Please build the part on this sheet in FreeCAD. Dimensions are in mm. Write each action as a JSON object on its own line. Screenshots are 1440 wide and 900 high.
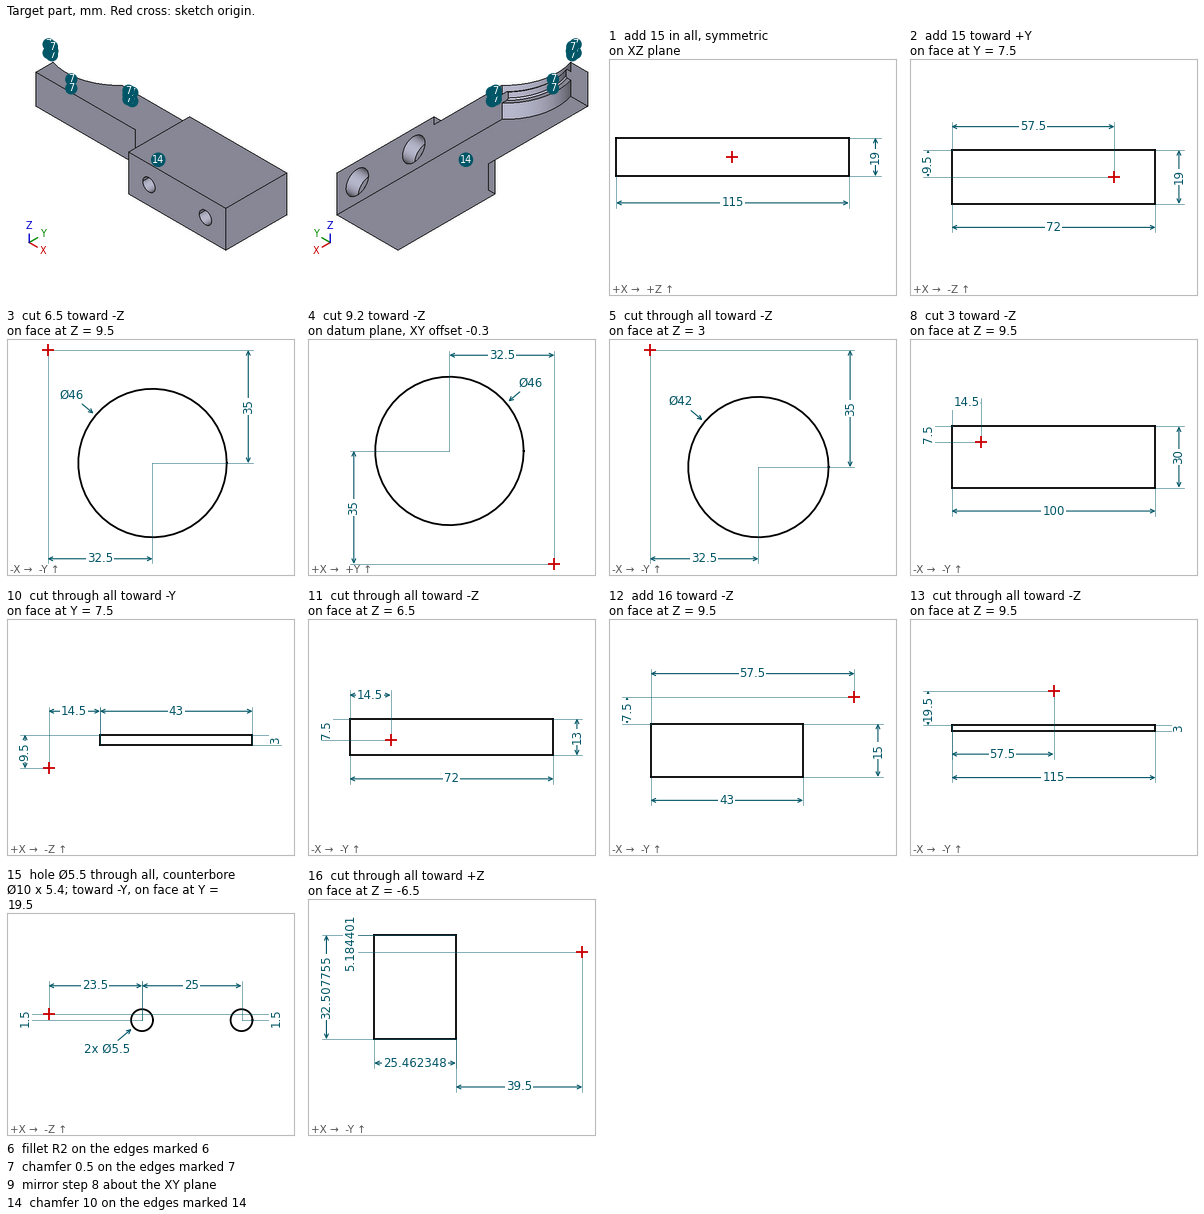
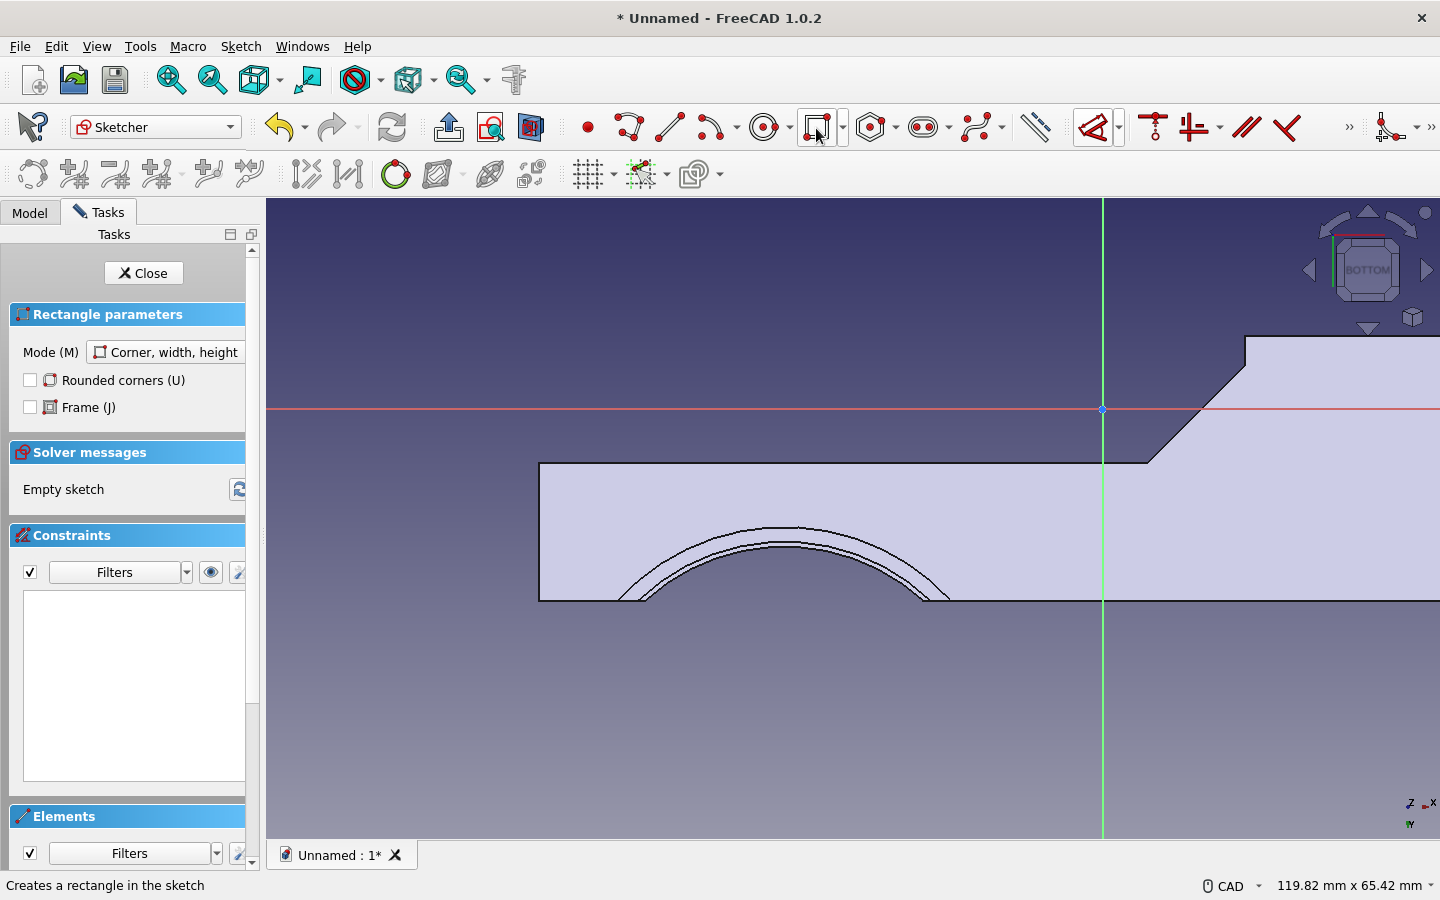
{"action": "left_click", "coordinate": [466, 359]}
{"action": "mouse_move", "coordinate": [716, 677]}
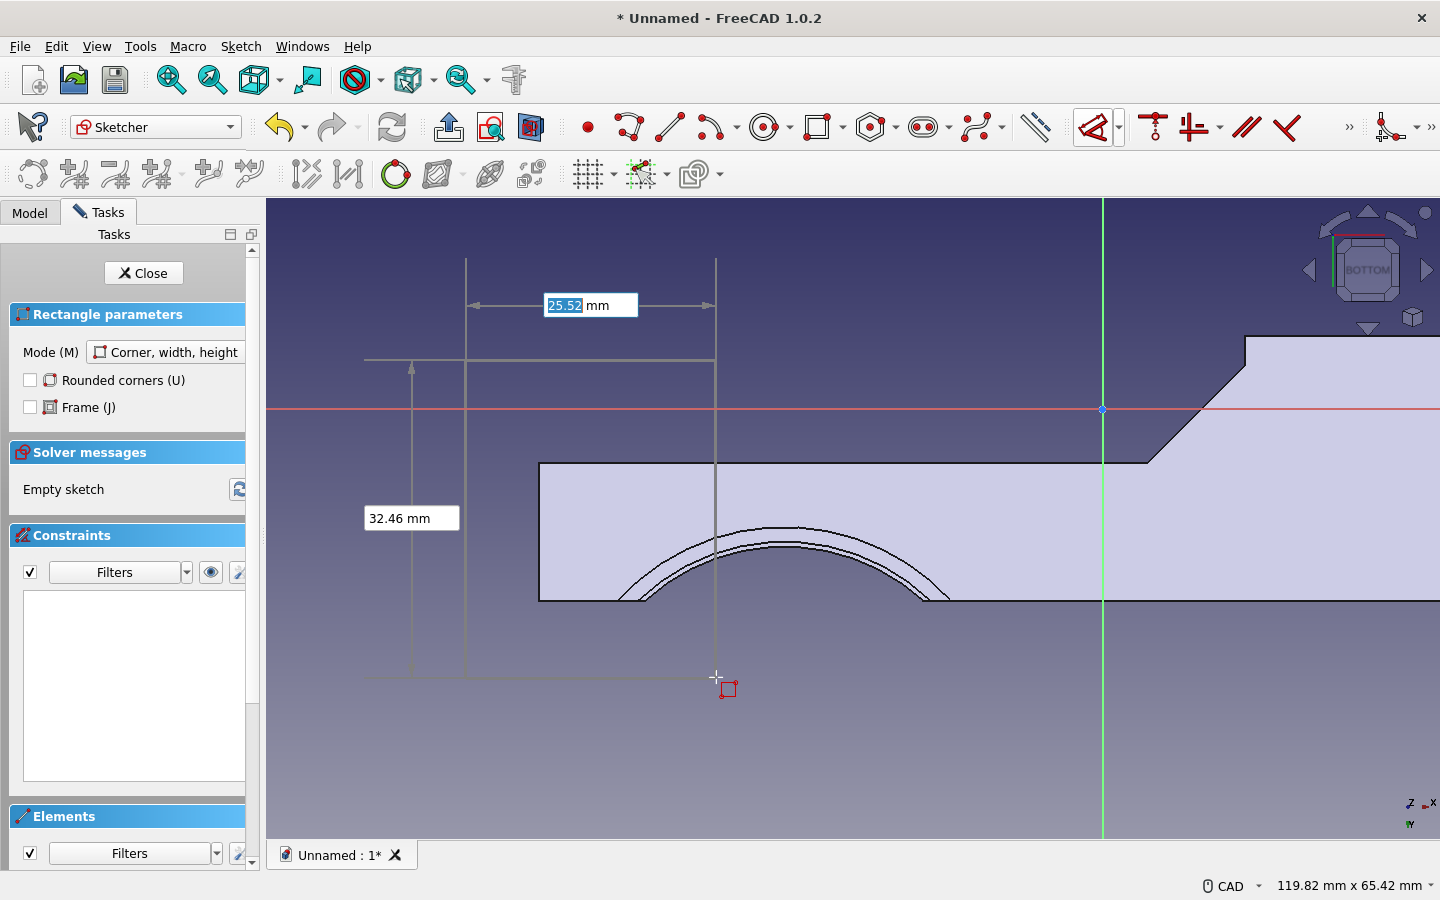
{"action": "type", "text": "25.462348"}
{"action": "key", "text": "Tab"}
{"action": "type", "text": "32.507755"}
{"action": "key", "text": "Return"}
{"action": "key", "text": "Escape"}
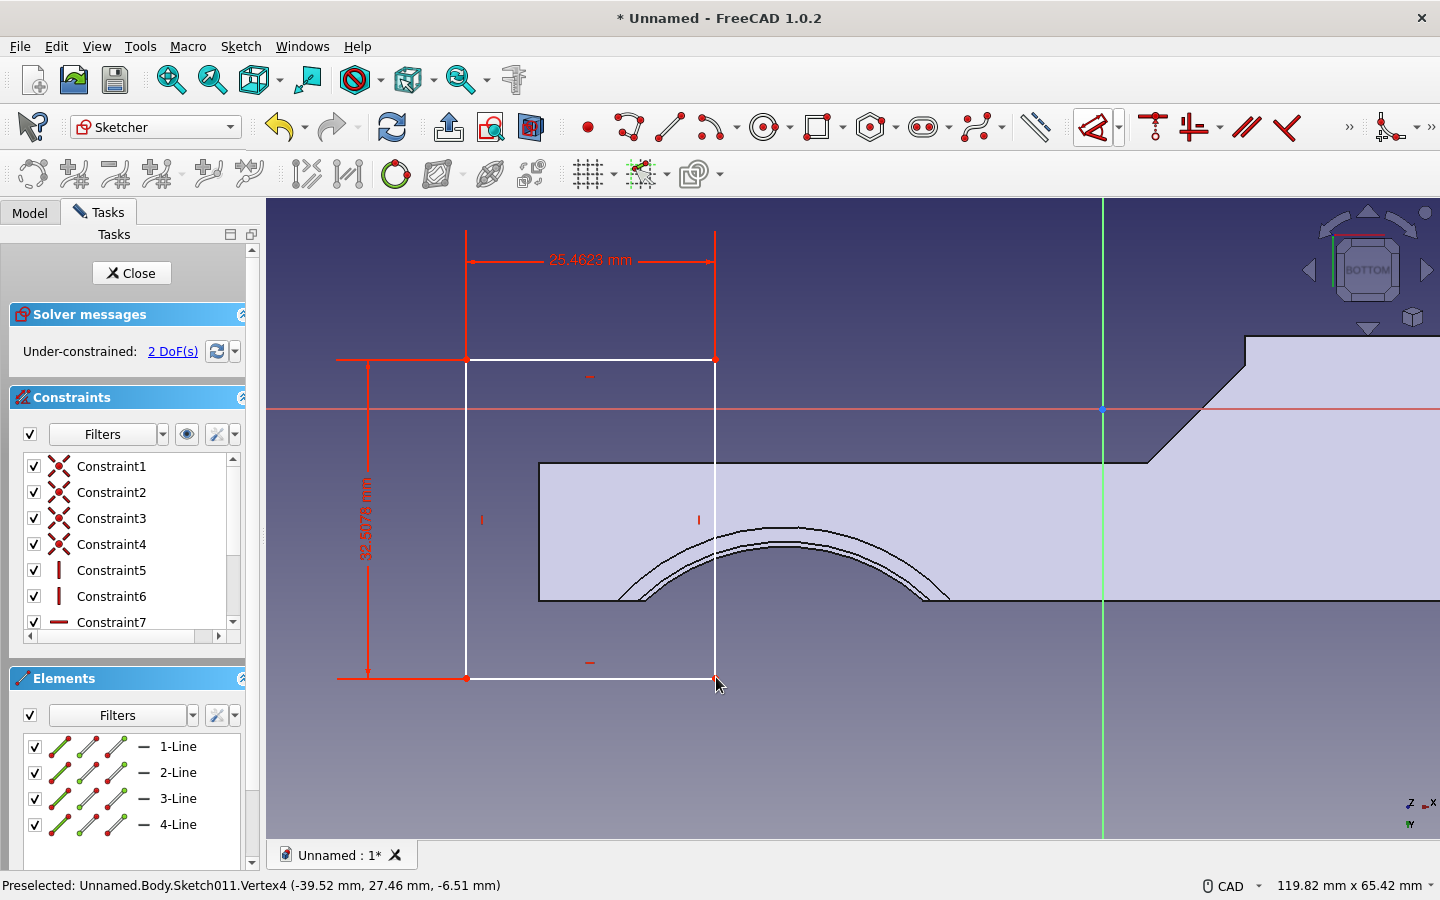
{"action": "left_click", "coordinate": [715, 679]}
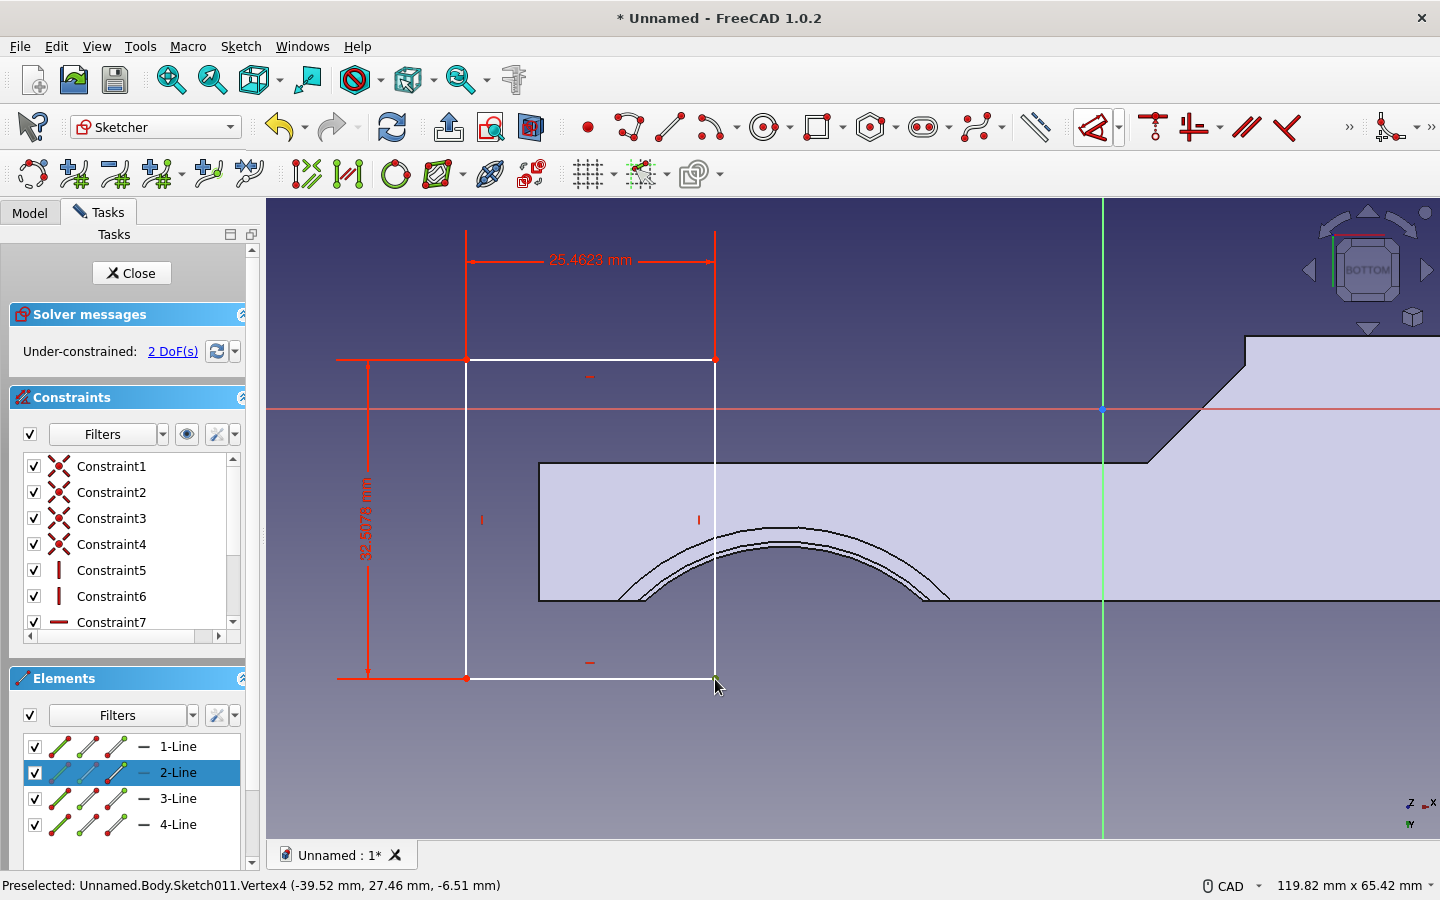
{"action": "left_click", "coordinate": [1118, 128]}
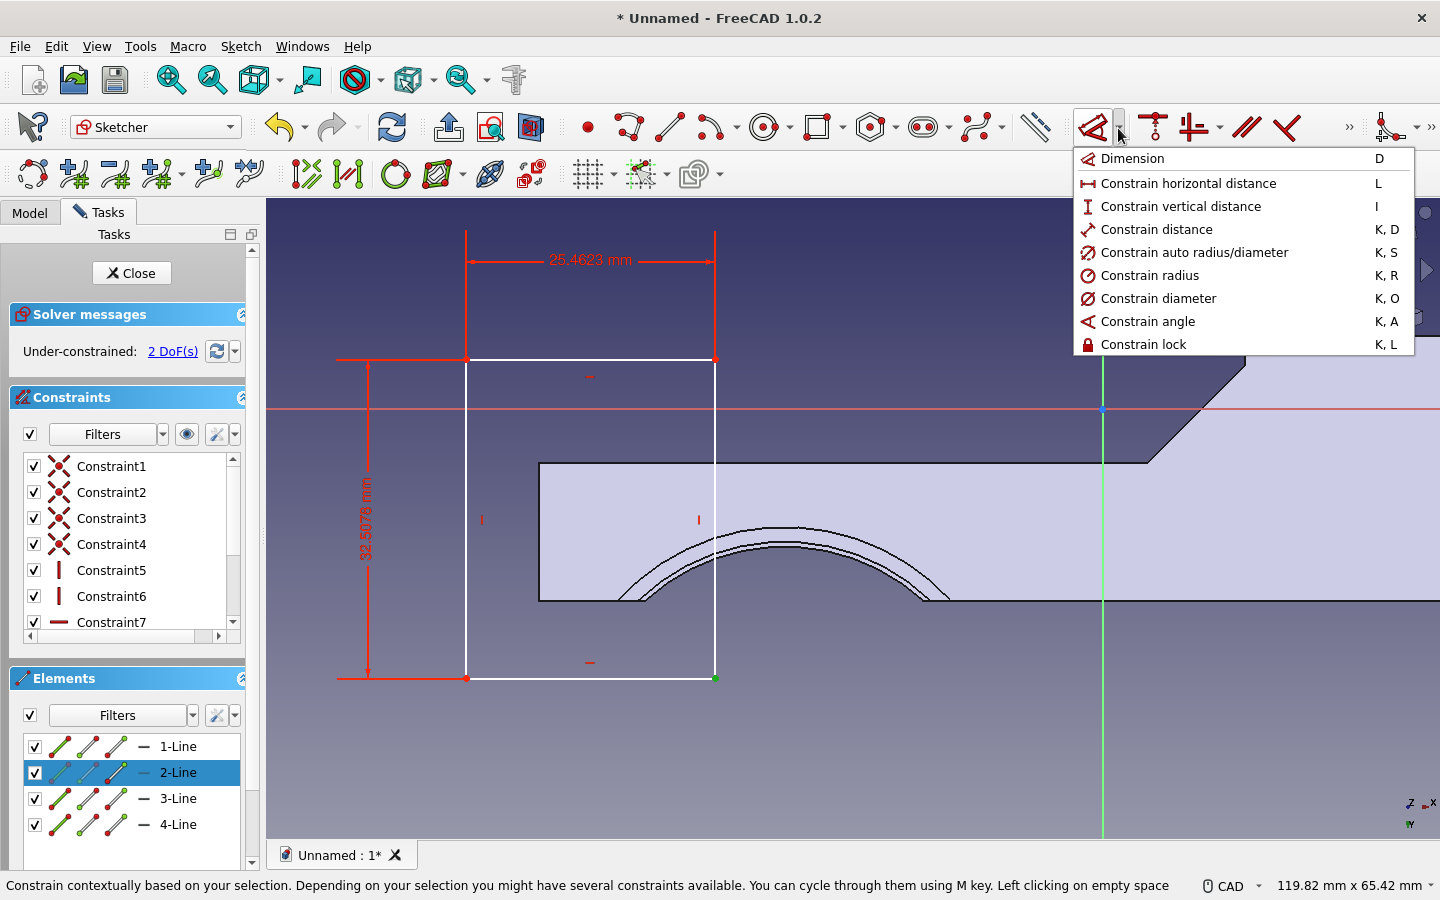
{"action": "left_click", "coordinate": [1244, 184]}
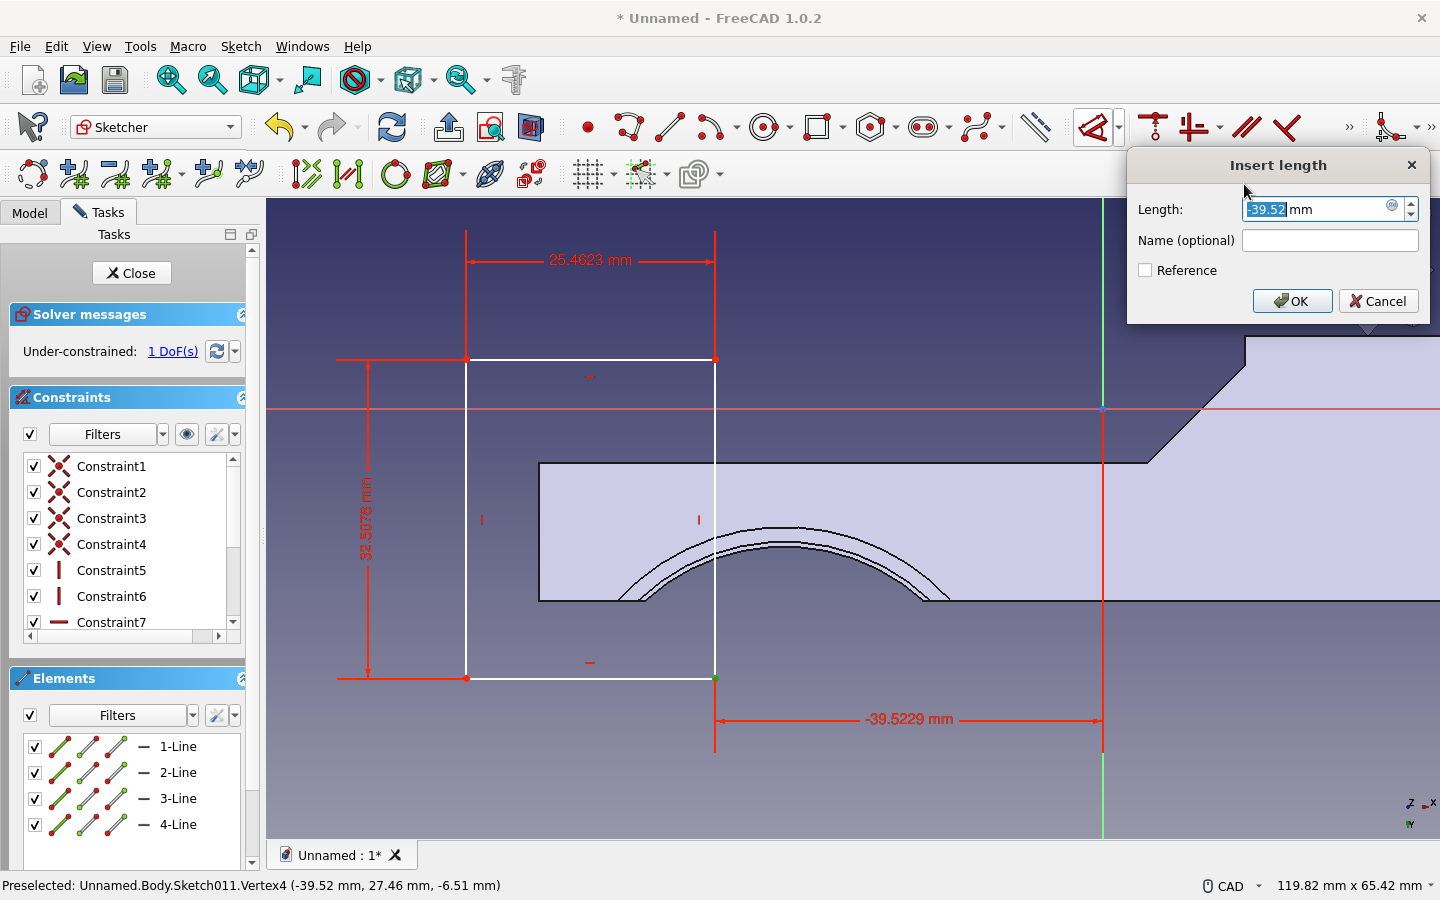
{"action": "type", "text": "-39.5"}
{"action": "key", "text": "Return"}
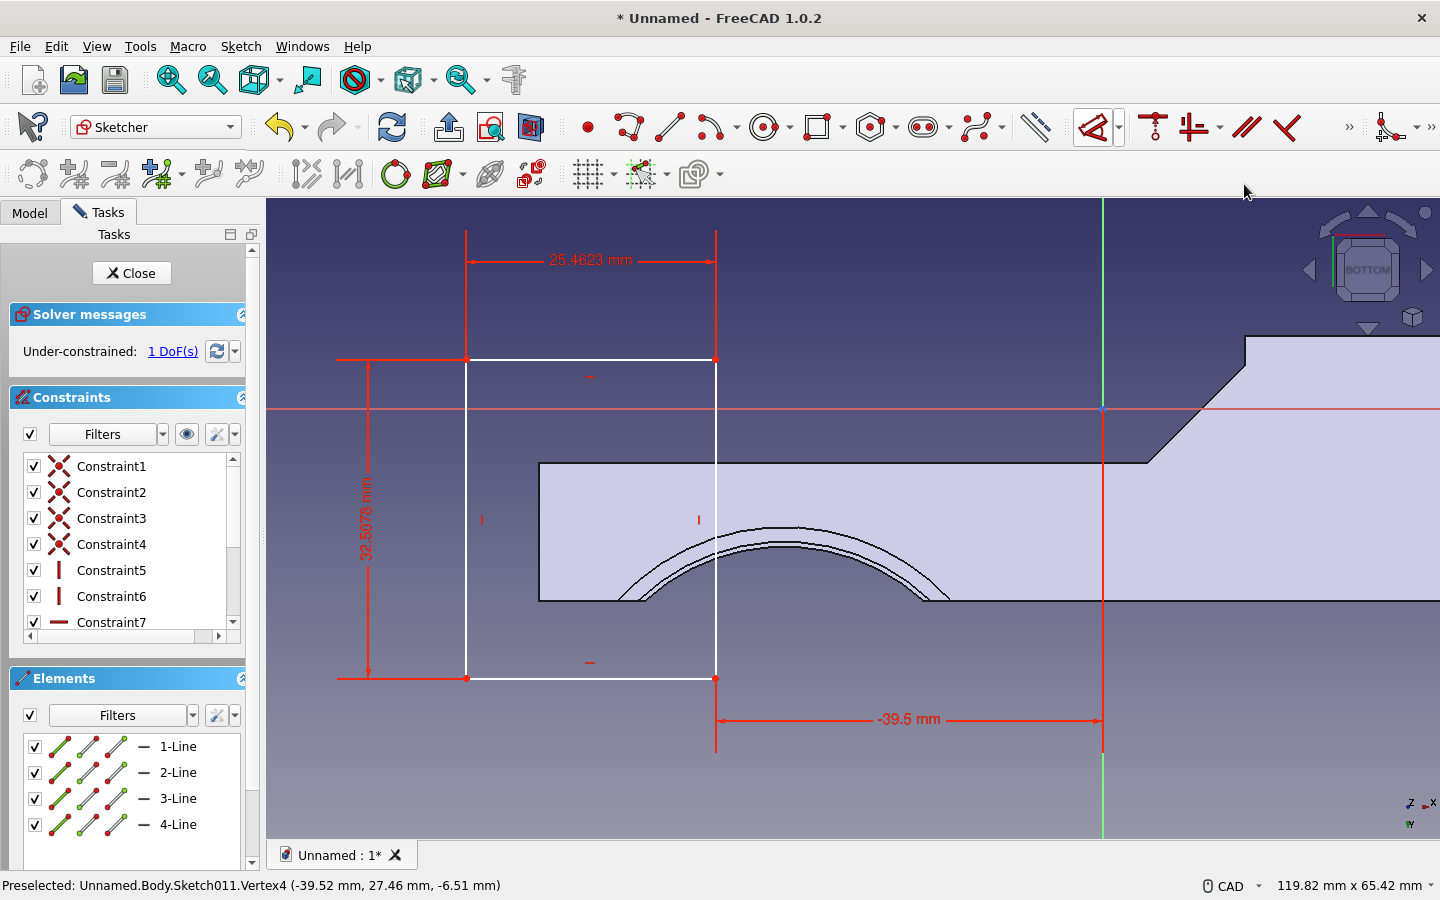
{"action": "left_click", "coordinate": [466, 360]}